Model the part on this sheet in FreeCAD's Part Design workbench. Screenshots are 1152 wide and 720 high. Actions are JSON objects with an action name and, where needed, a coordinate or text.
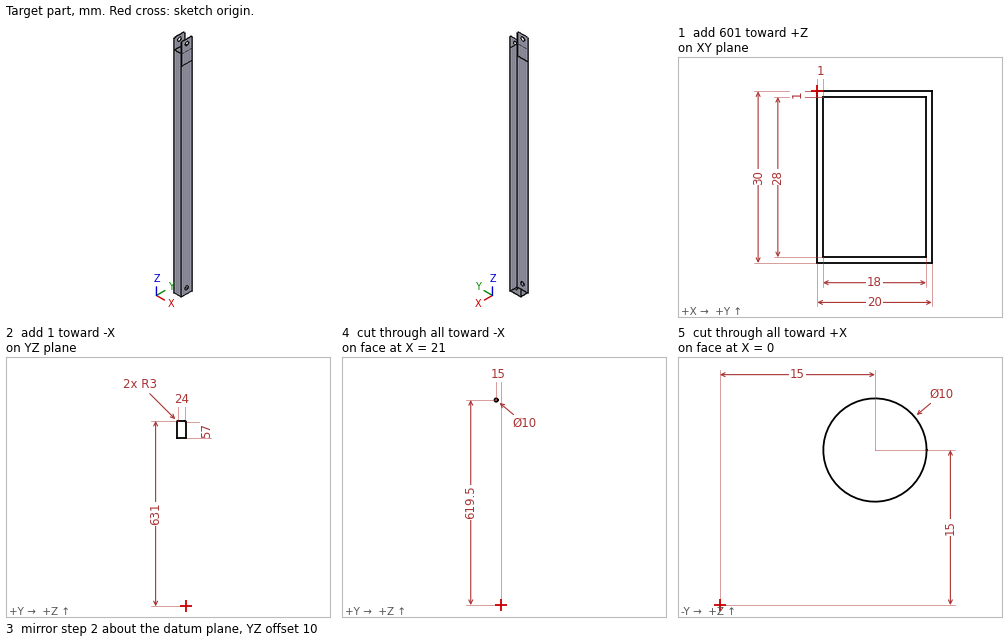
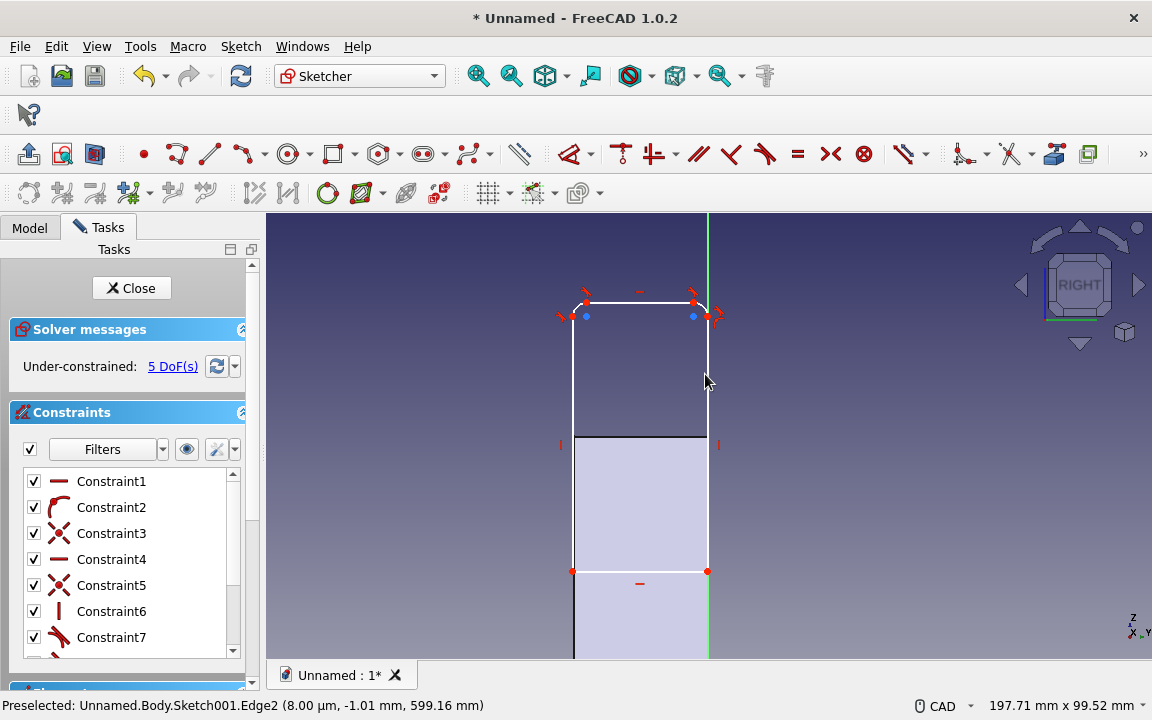
{"action": "scroll", "coordinate": [700, 304], "scroll_direction": "up", "scroll_amount": 4}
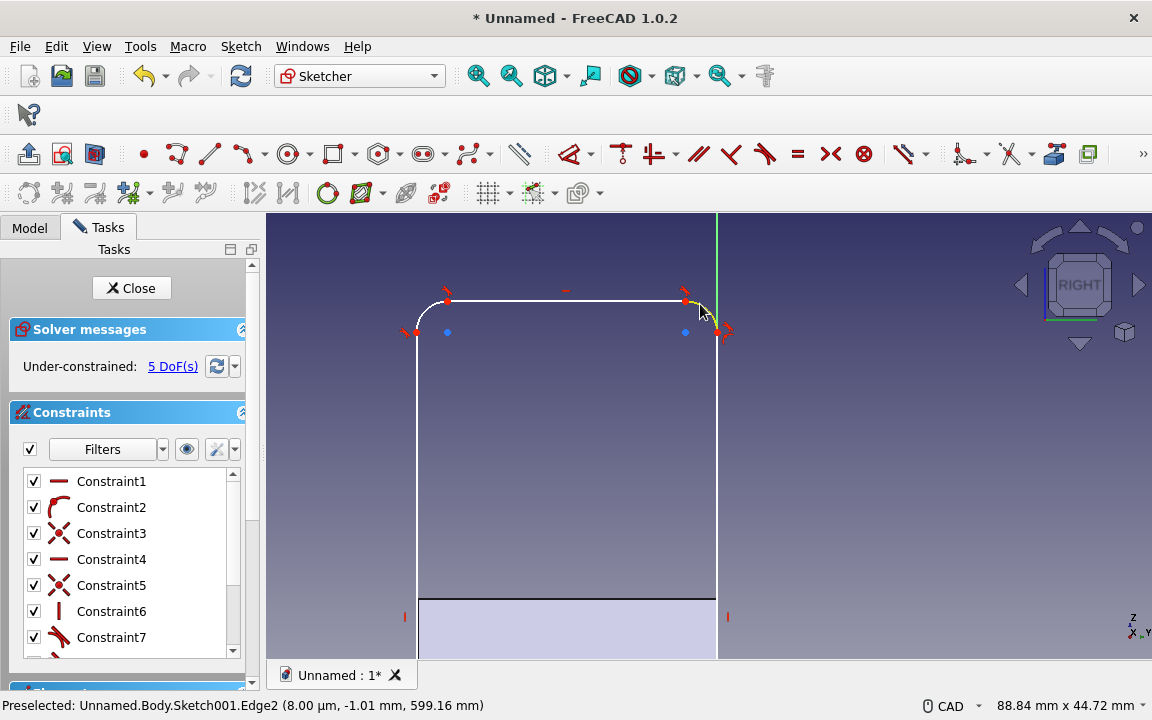
{"action": "left_click", "coordinate": [700, 305]}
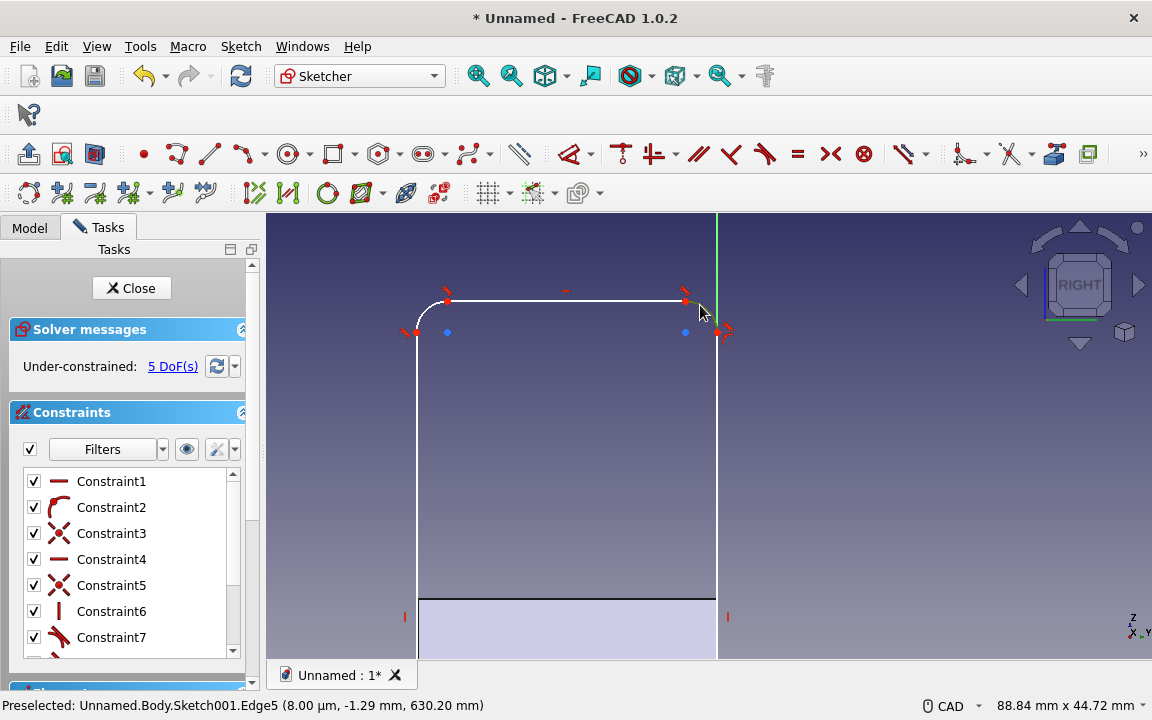
{"action": "left_click", "coordinate": [434, 305]}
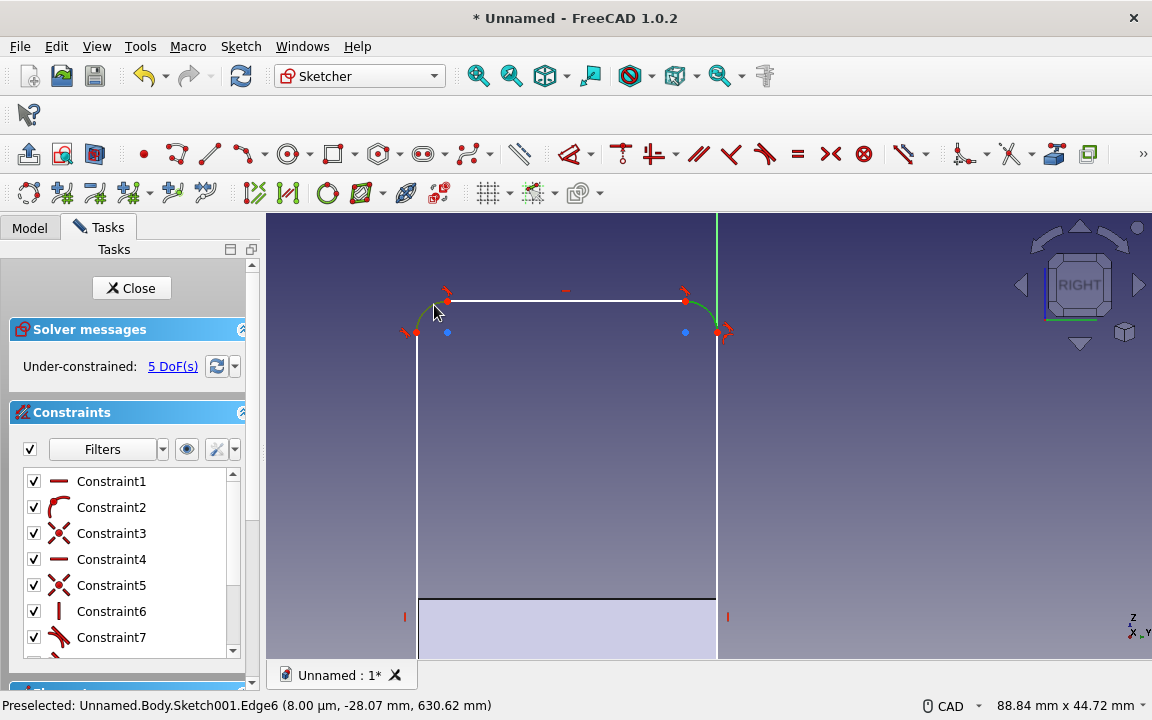
{"action": "key", "text": "e"}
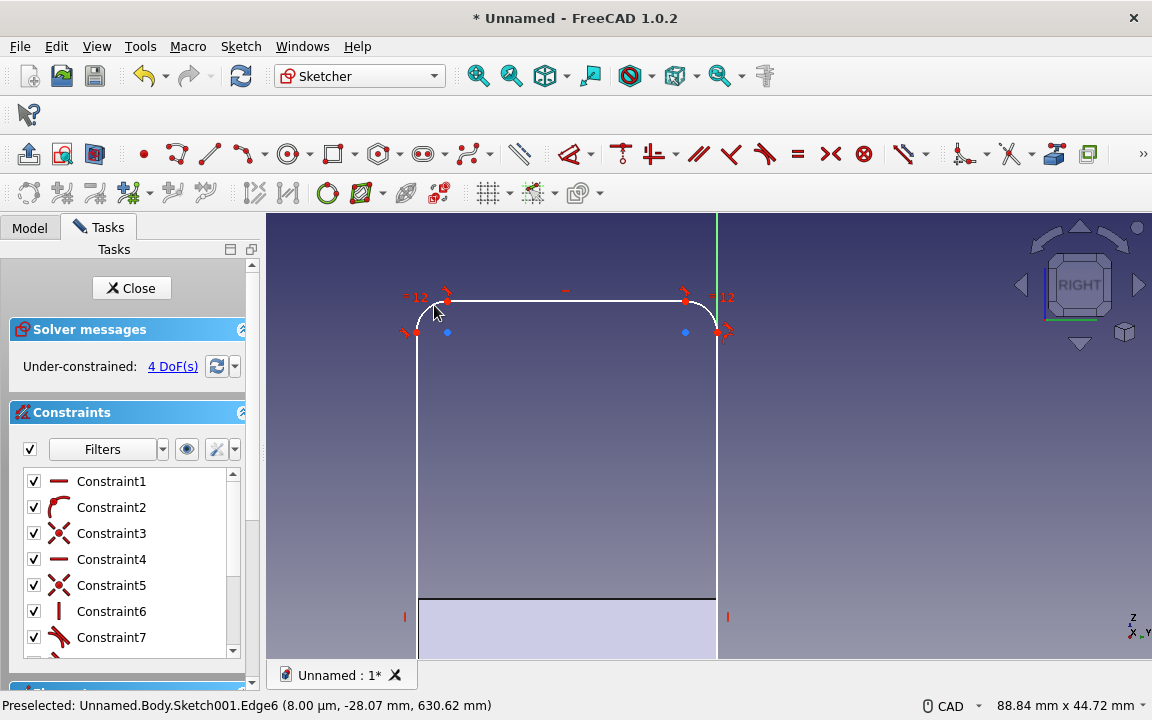
{"action": "key", "text": "d"}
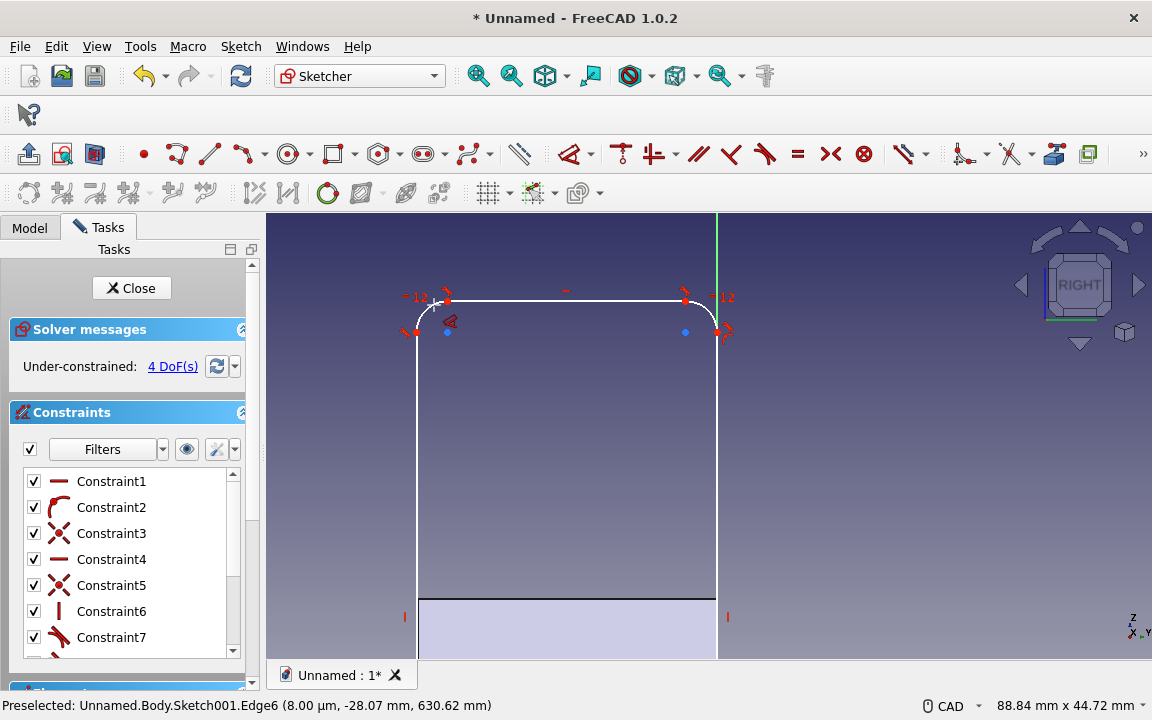
{"action": "scroll", "coordinate": [714, 318], "scroll_direction": "up", "scroll_amount": 2}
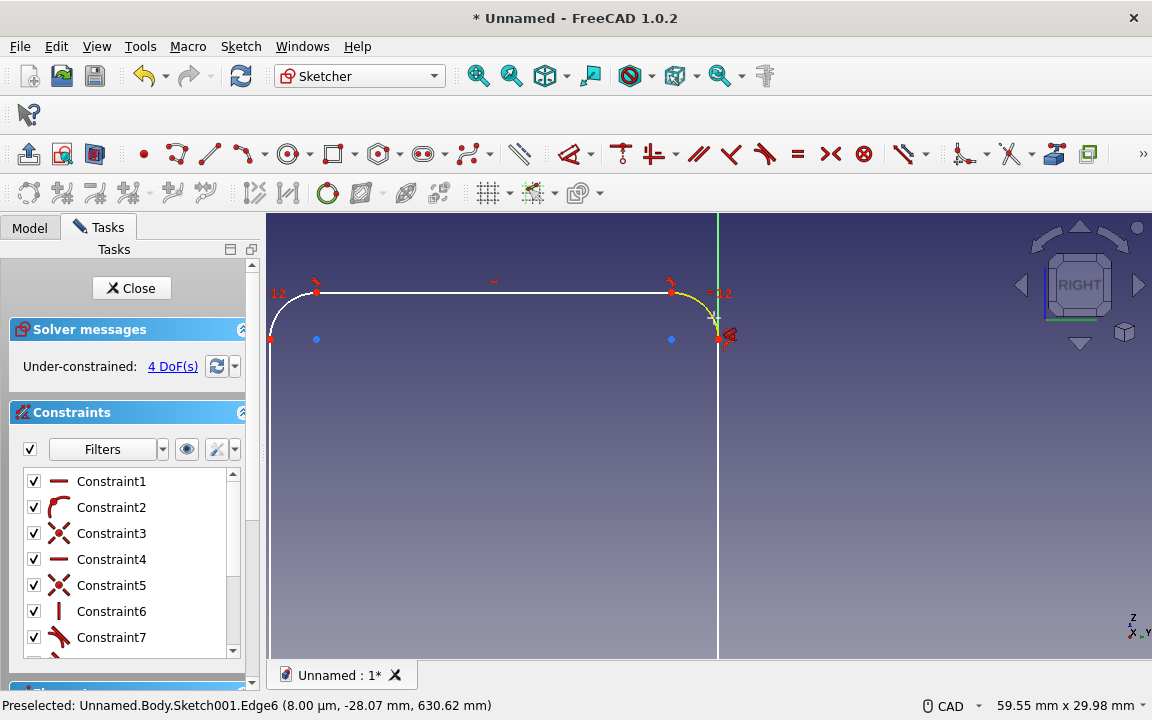
{"action": "left_click", "coordinate": [713, 318]}
{"action": "left_click", "coordinate": [741, 303]}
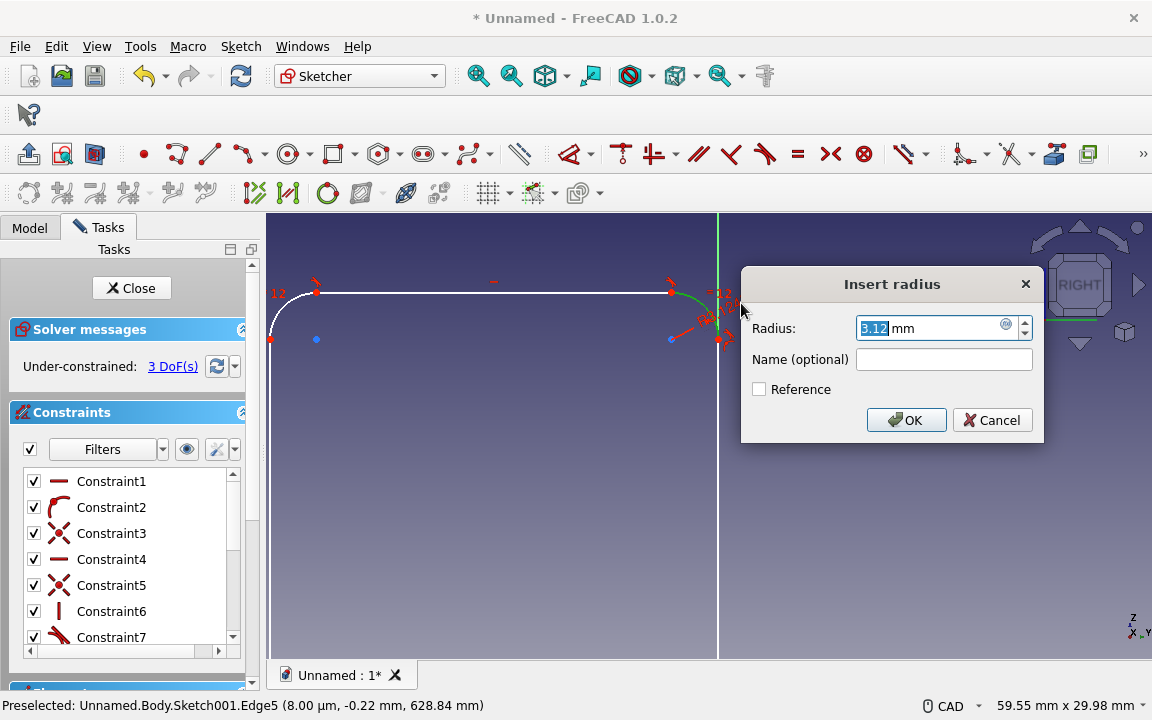
{"action": "type", "text": "3"}
{"action": "key", "text": "Return"}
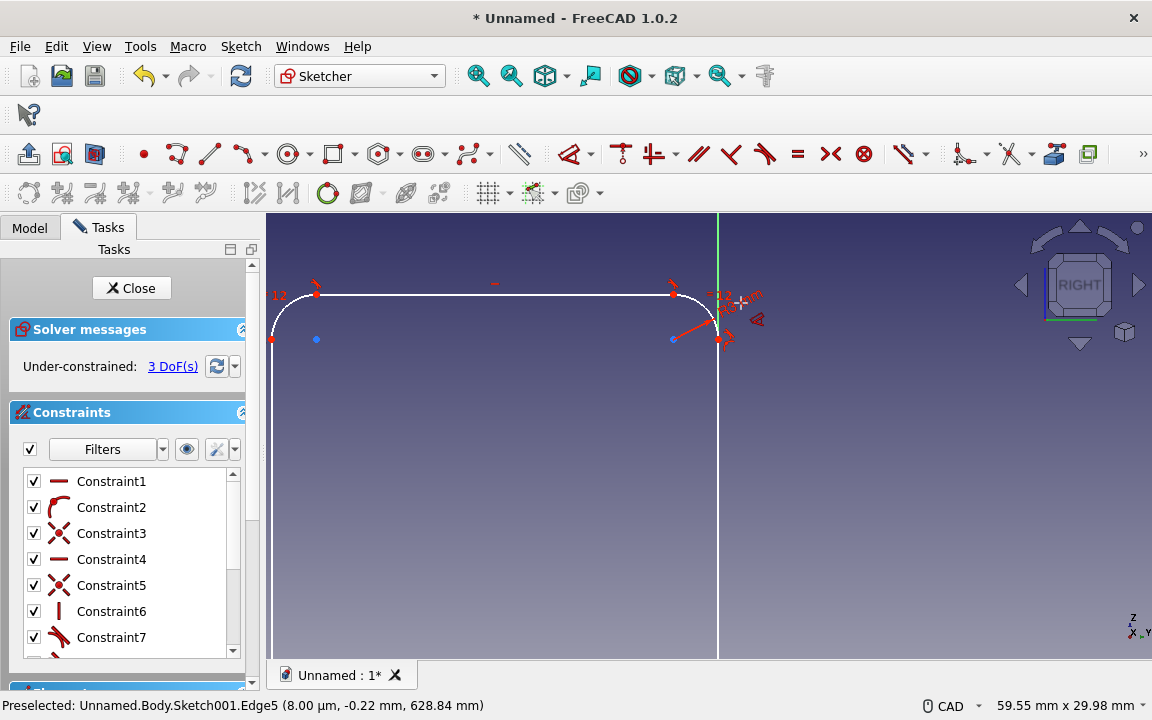
{"action": "left_click", "coordinate": [424, 295]}
{"action": "left_click", "coordinate": [495, 261]}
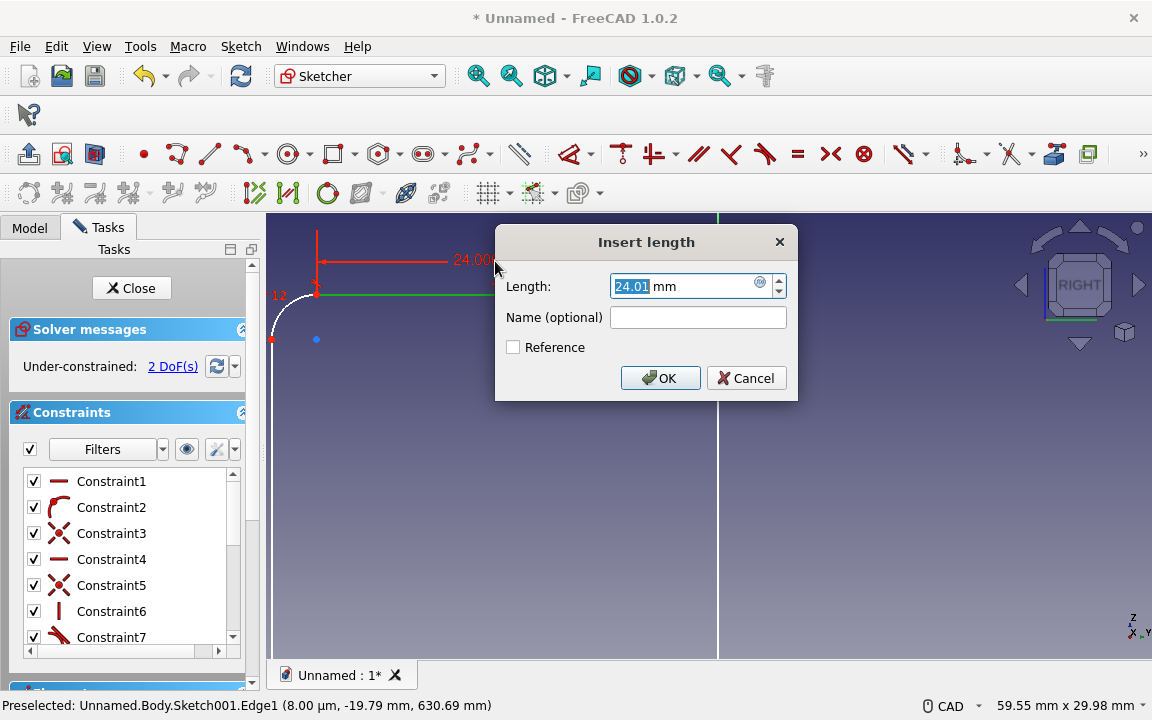
{"action": "type", "text": "24"}
{"action": "key", "text": "Return"}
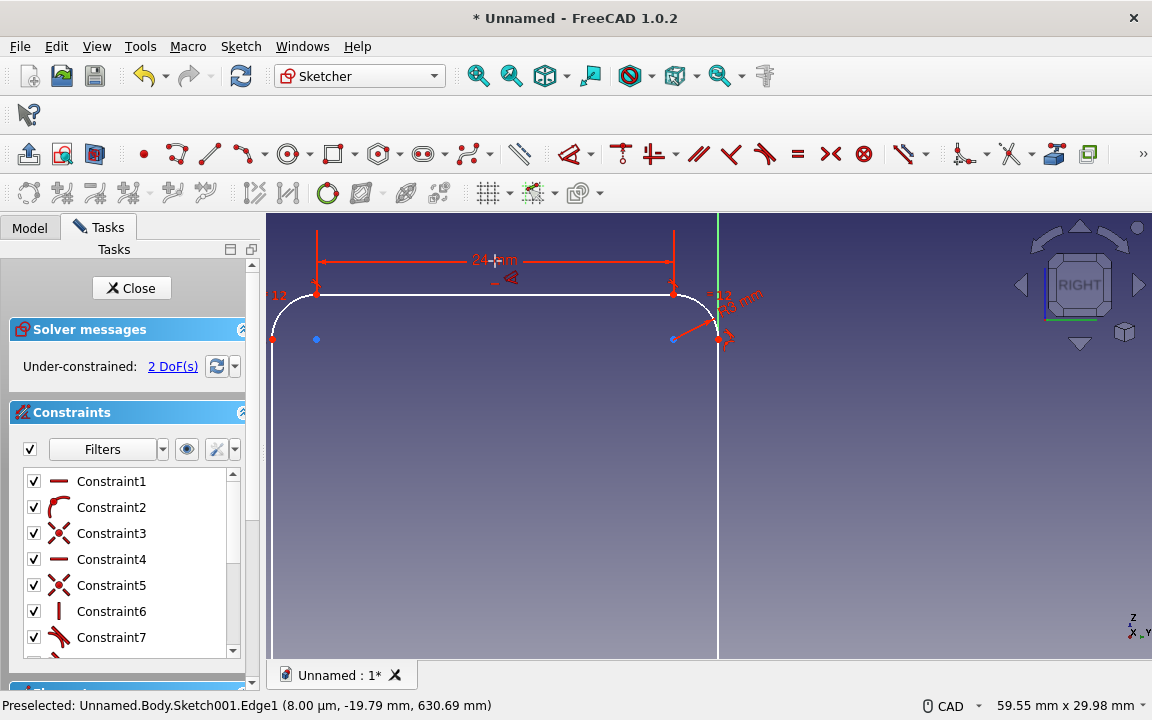
{"action": "left_click", "coordinate": [718, 594]}
{"action": "left_click", "coordinate": [752, 485]}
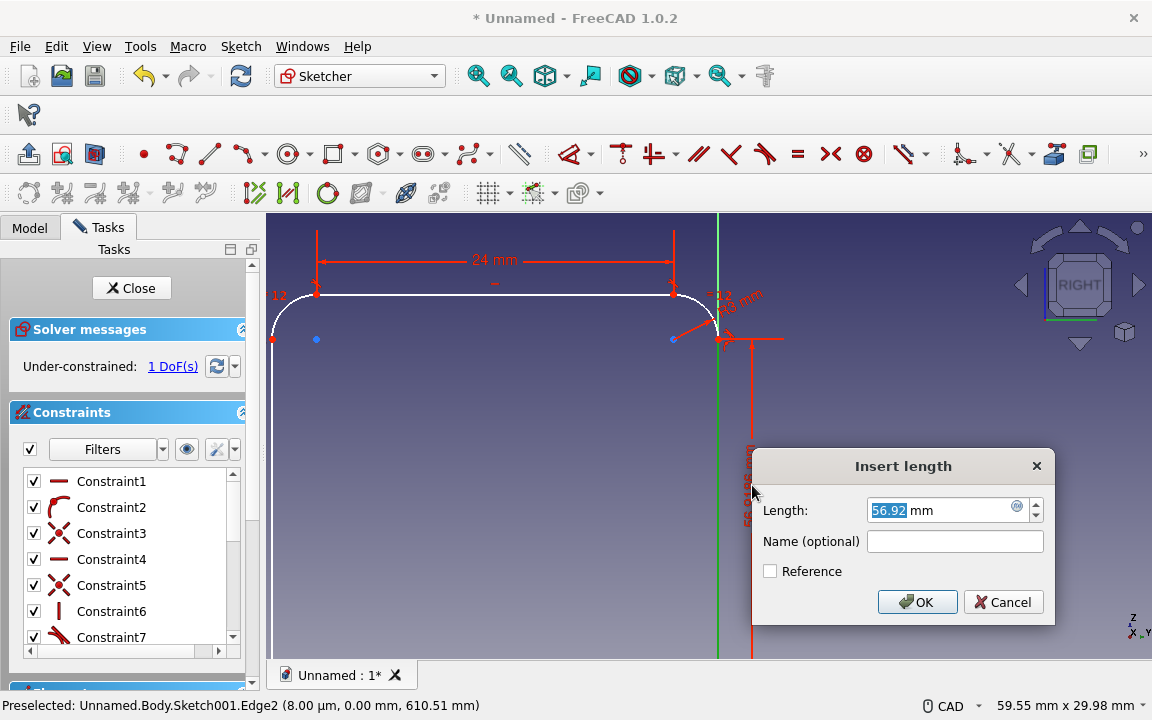
{"action": "type", "text": "57"}
{"action": "key", "text": "Return"}